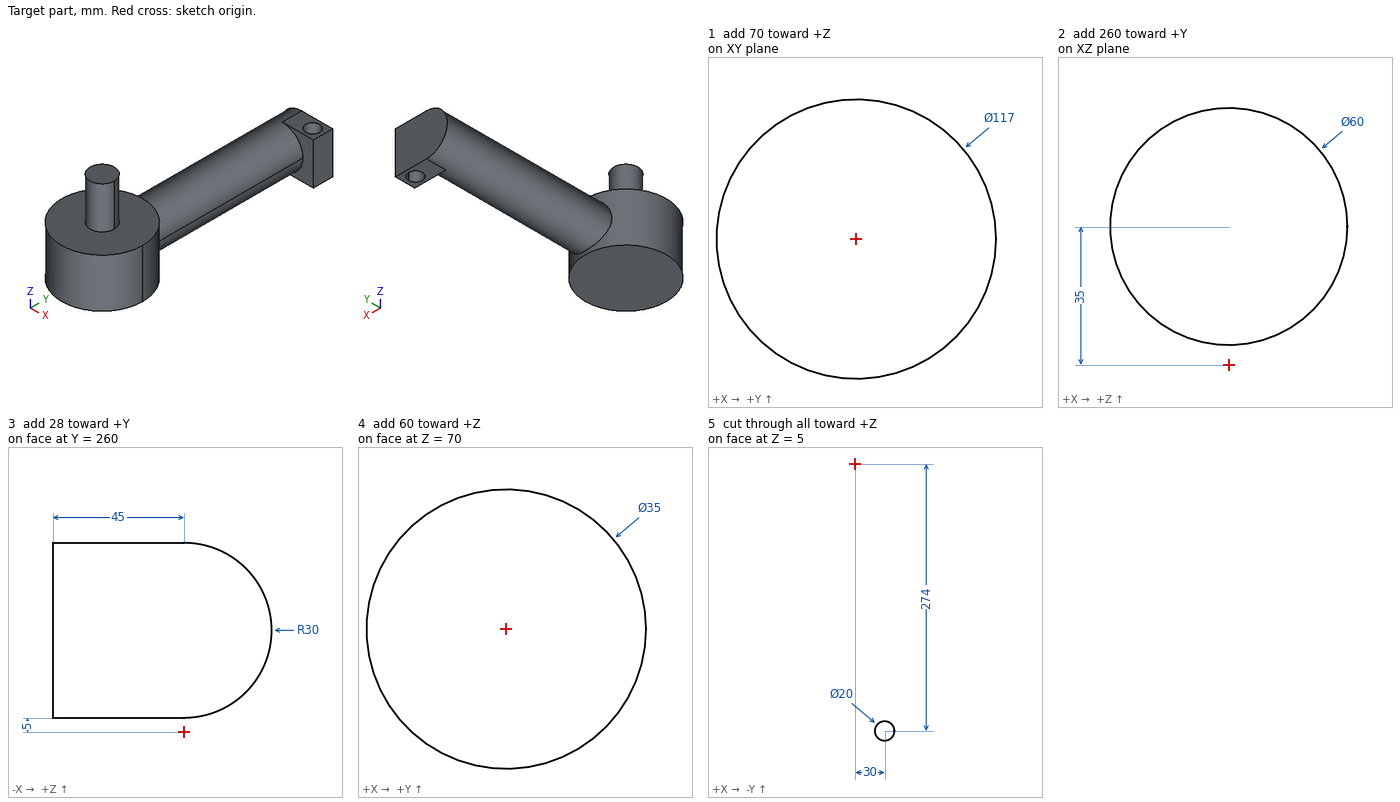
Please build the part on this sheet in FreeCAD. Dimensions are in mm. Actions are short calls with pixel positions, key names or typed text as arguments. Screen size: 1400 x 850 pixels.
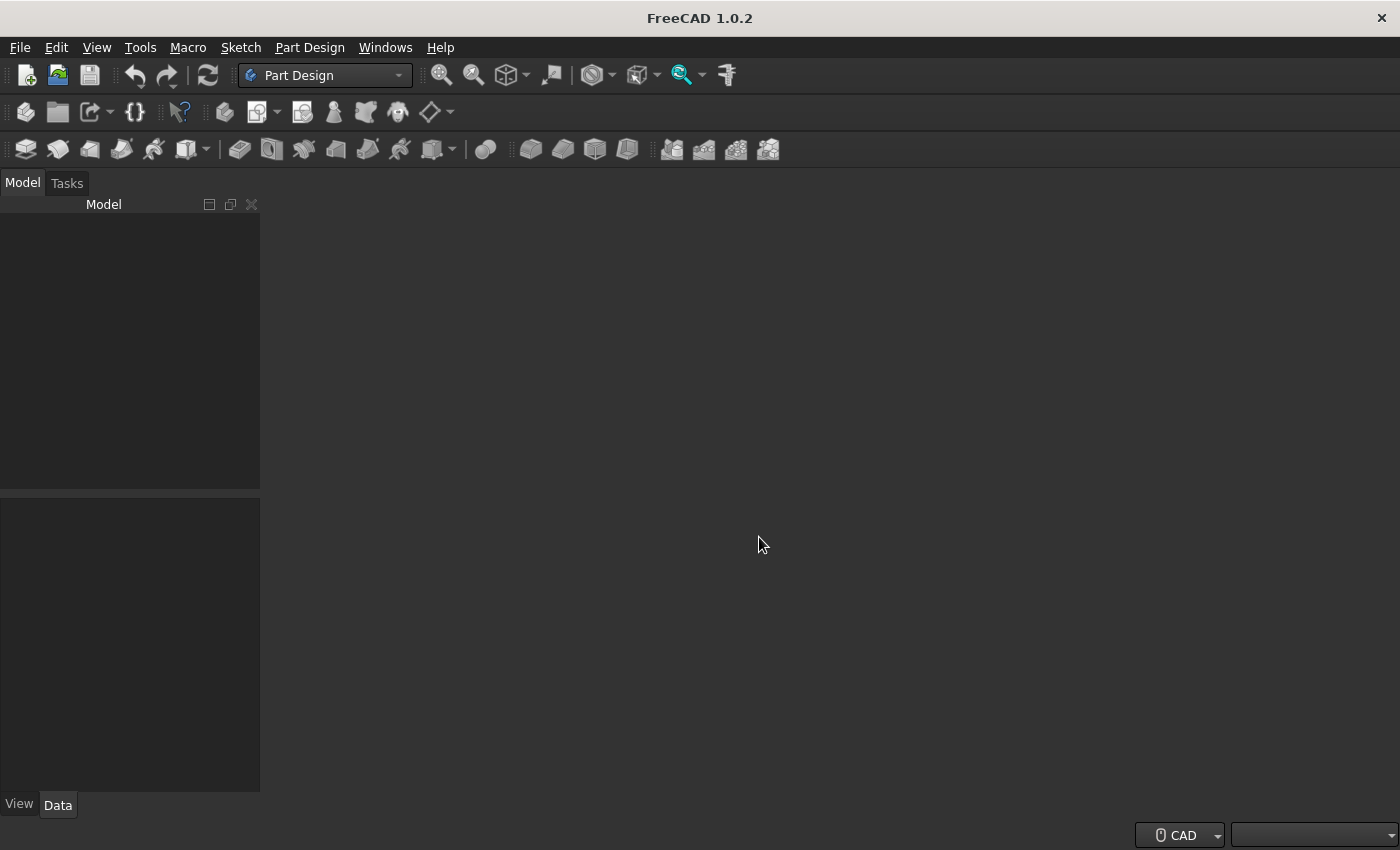
click(26, 76)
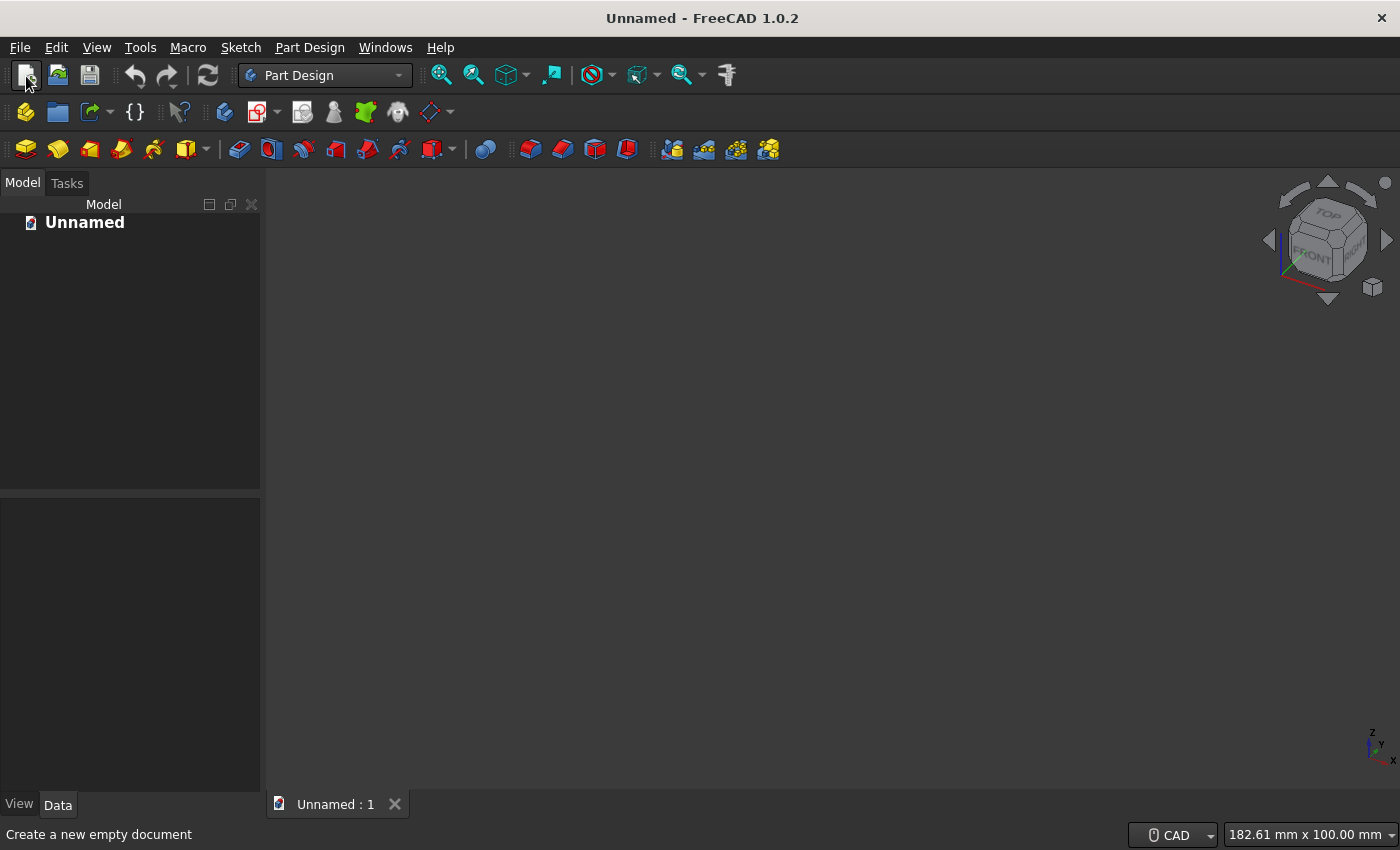
click(258, 112)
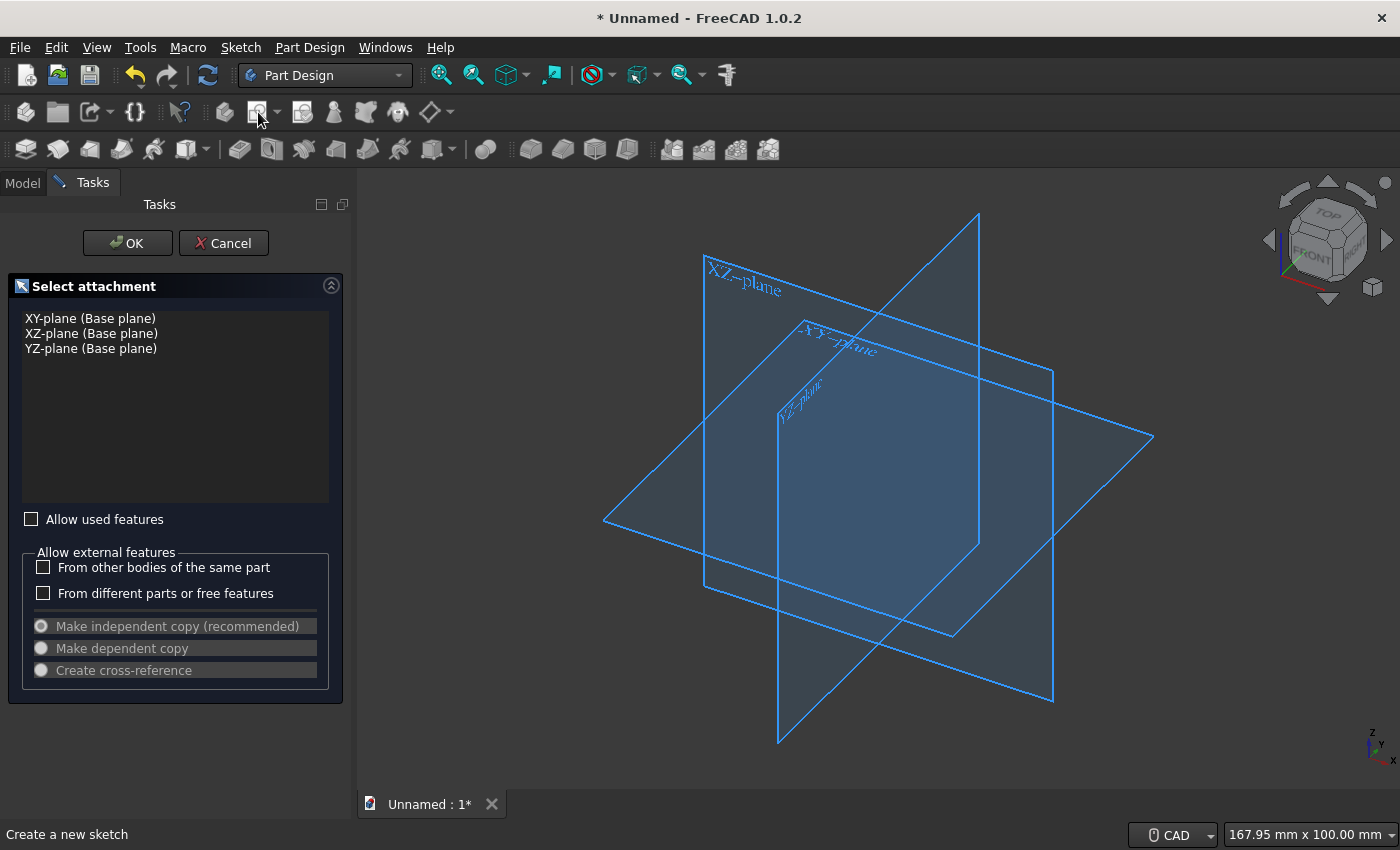
click(82, 318)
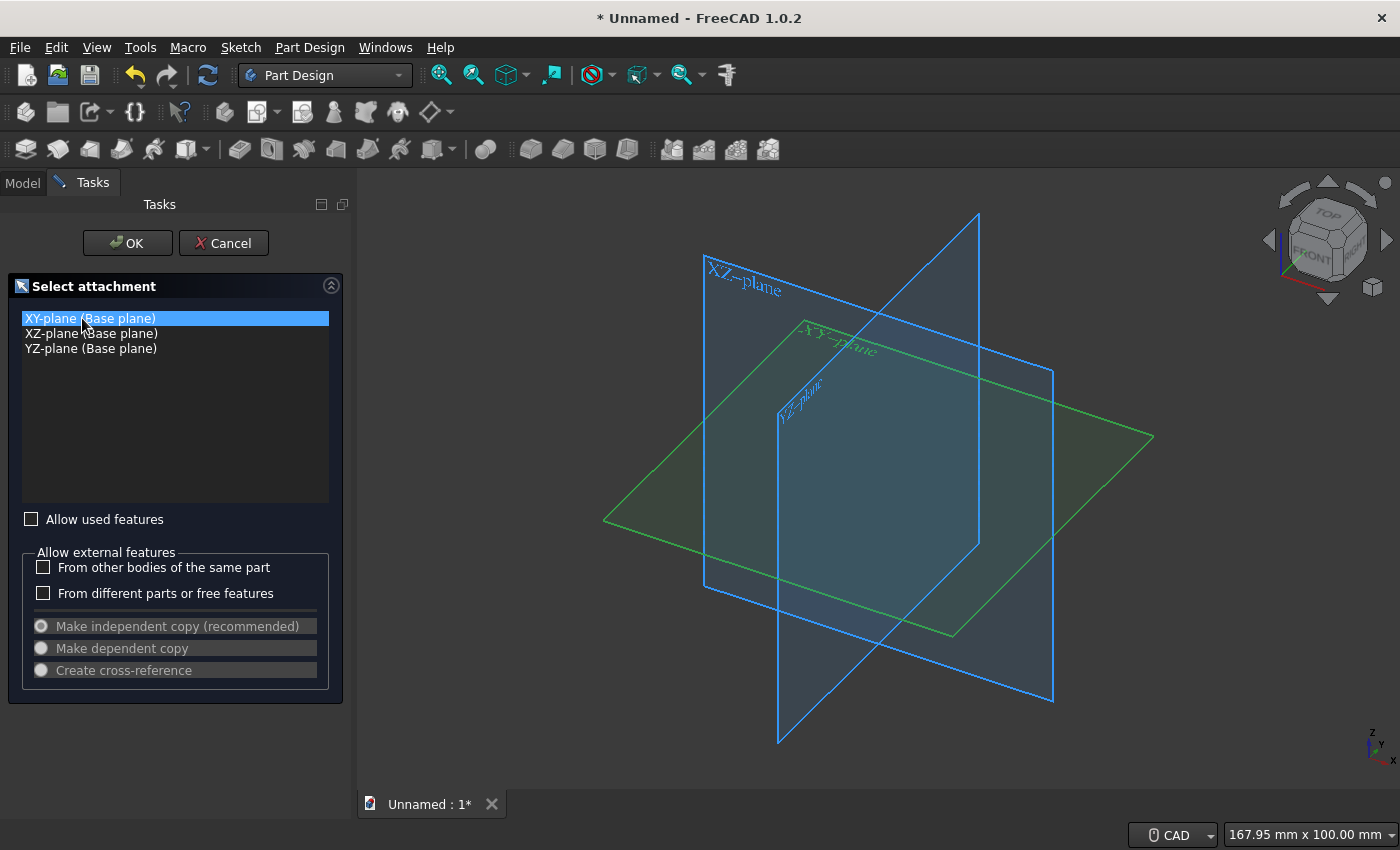
click(128, 243)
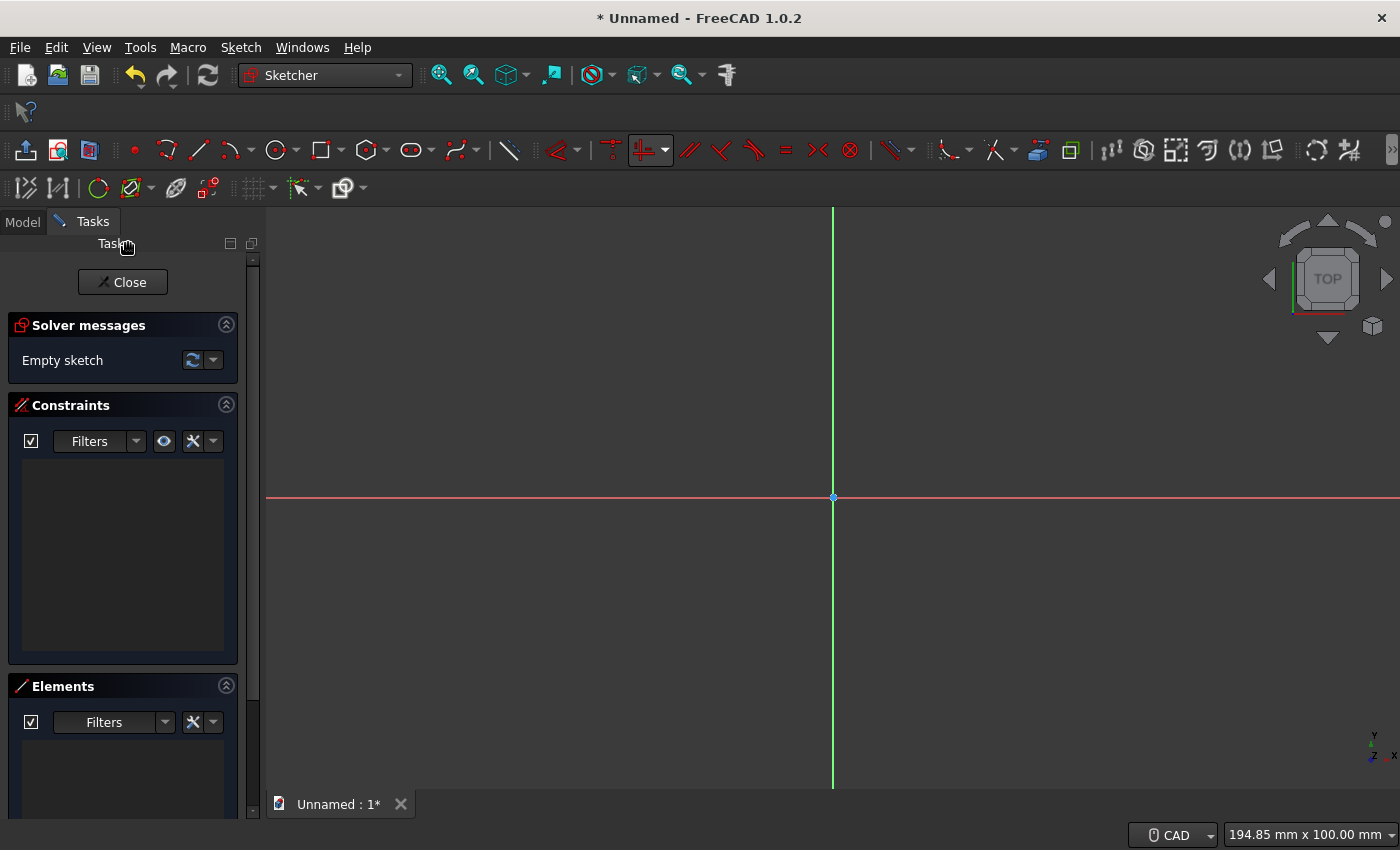
scroll(681, 498, down, 3)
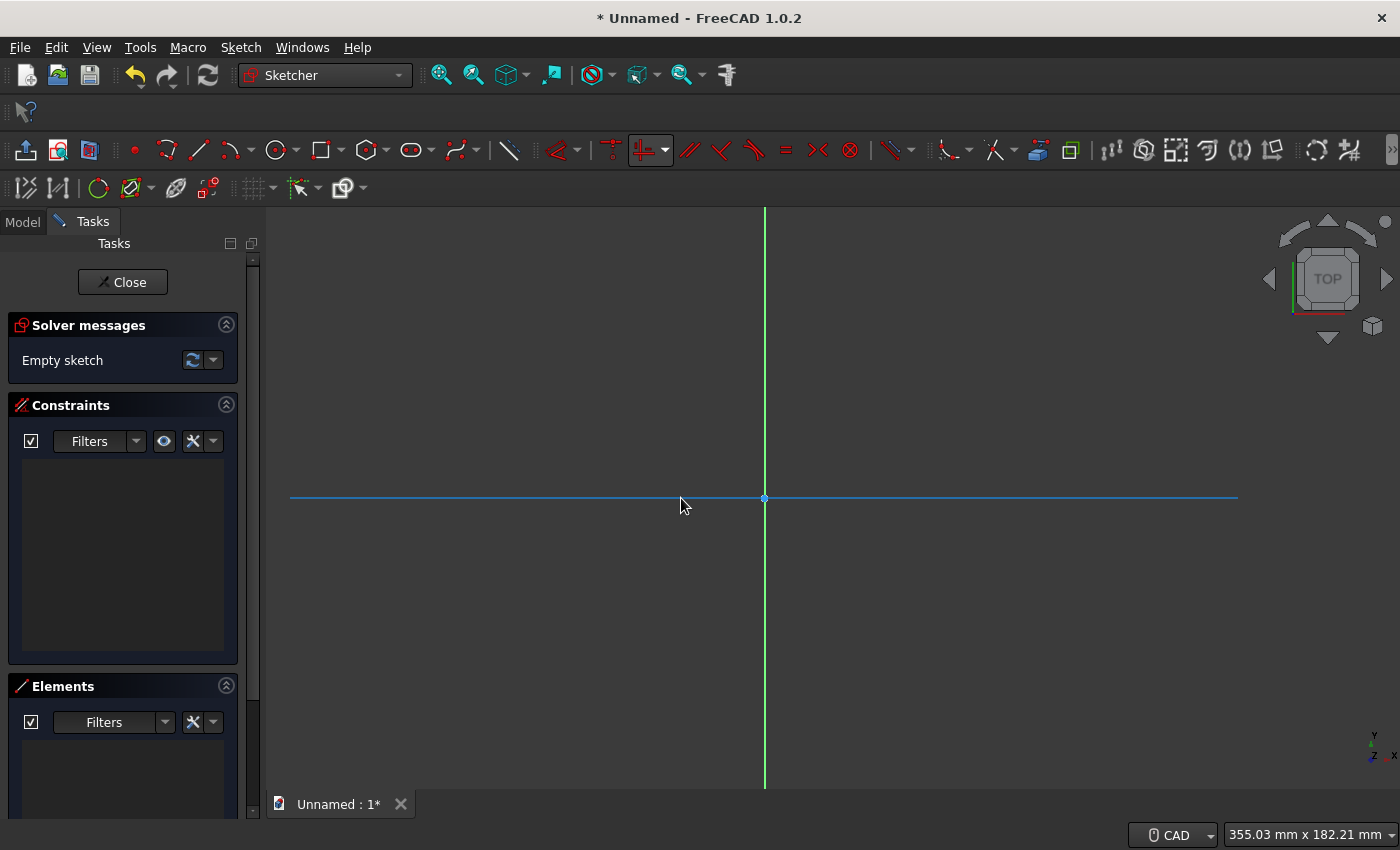
click(276, 150)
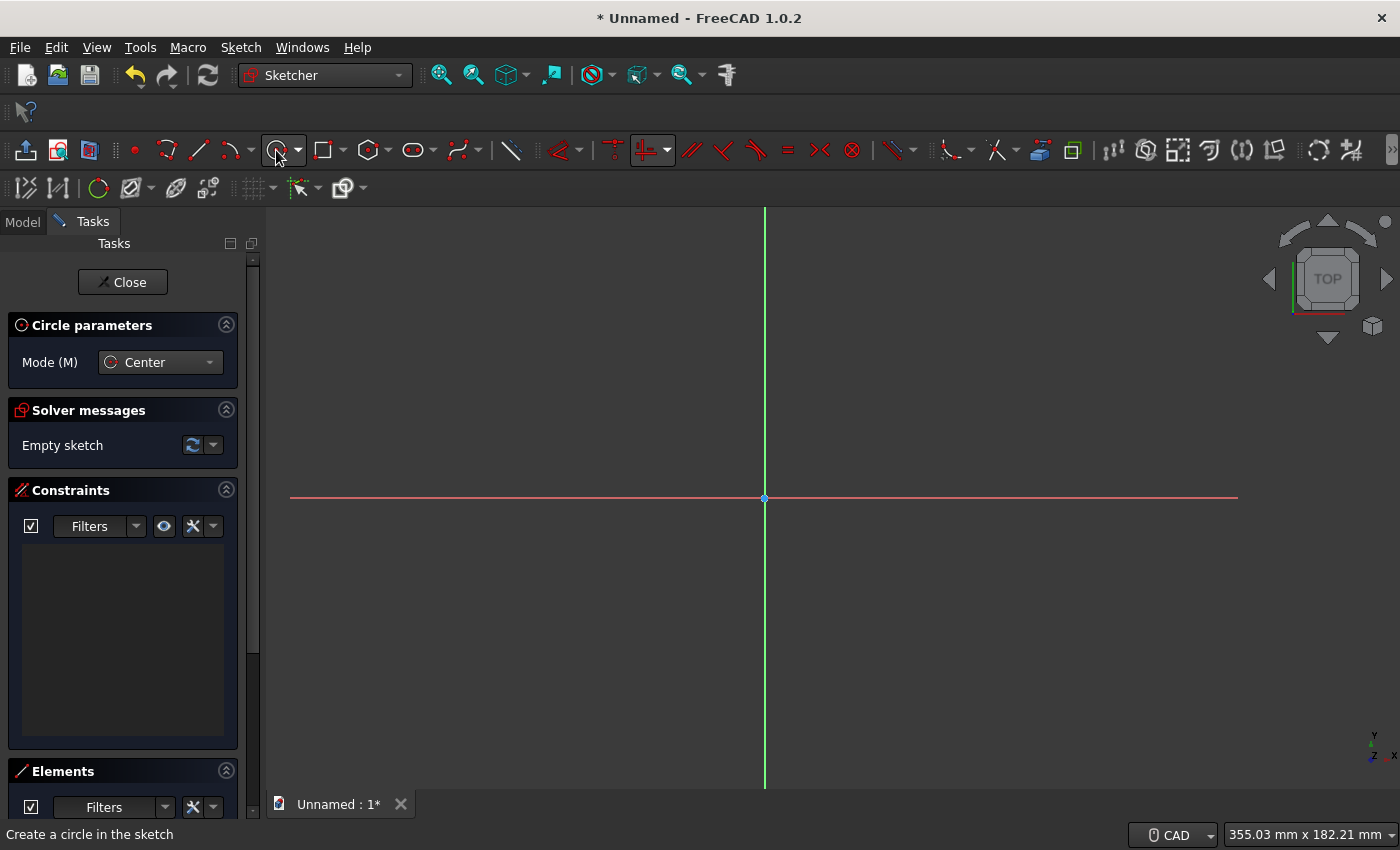
click(765, 498)
click(897, 366)
key(Escape)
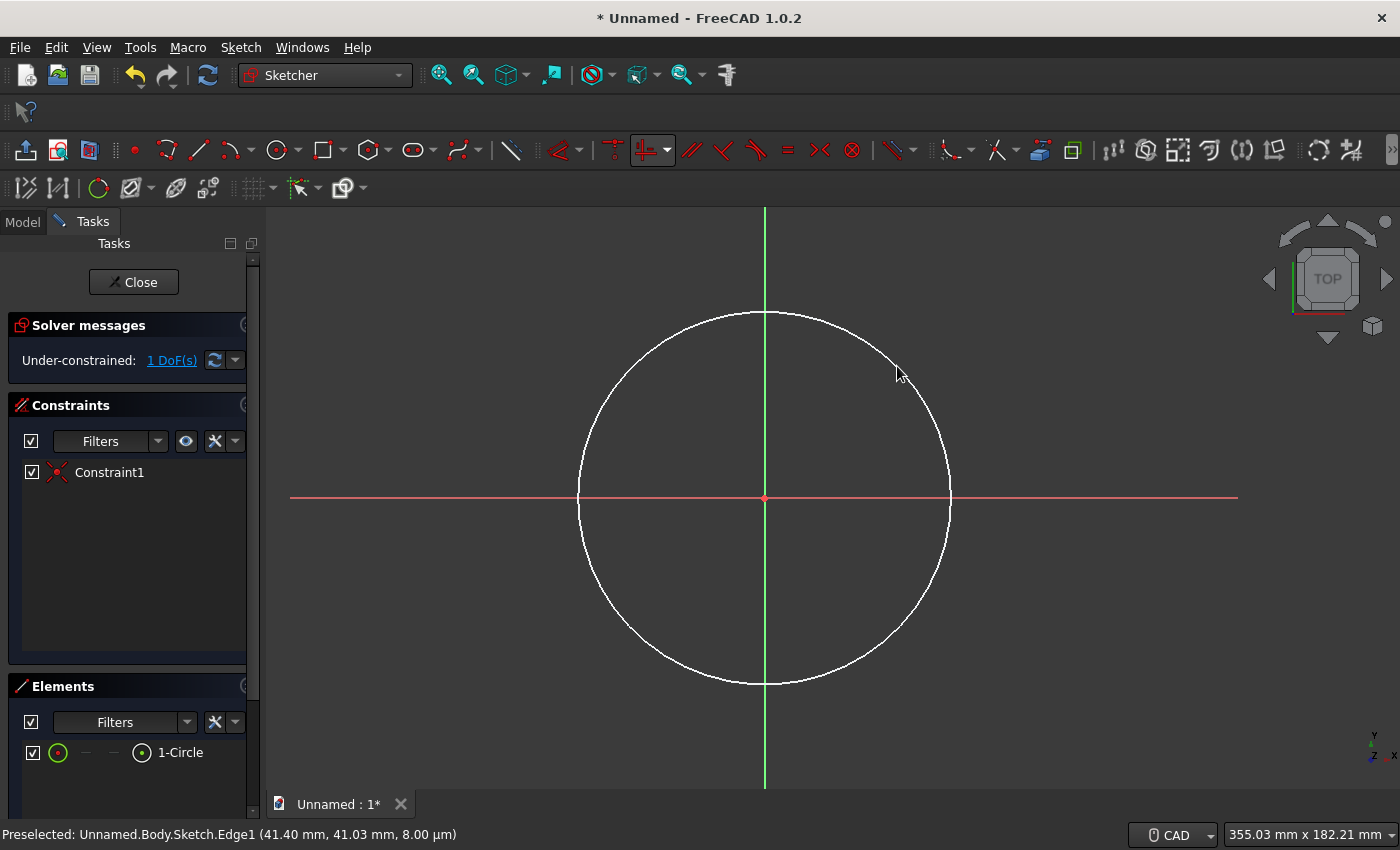
key(d)